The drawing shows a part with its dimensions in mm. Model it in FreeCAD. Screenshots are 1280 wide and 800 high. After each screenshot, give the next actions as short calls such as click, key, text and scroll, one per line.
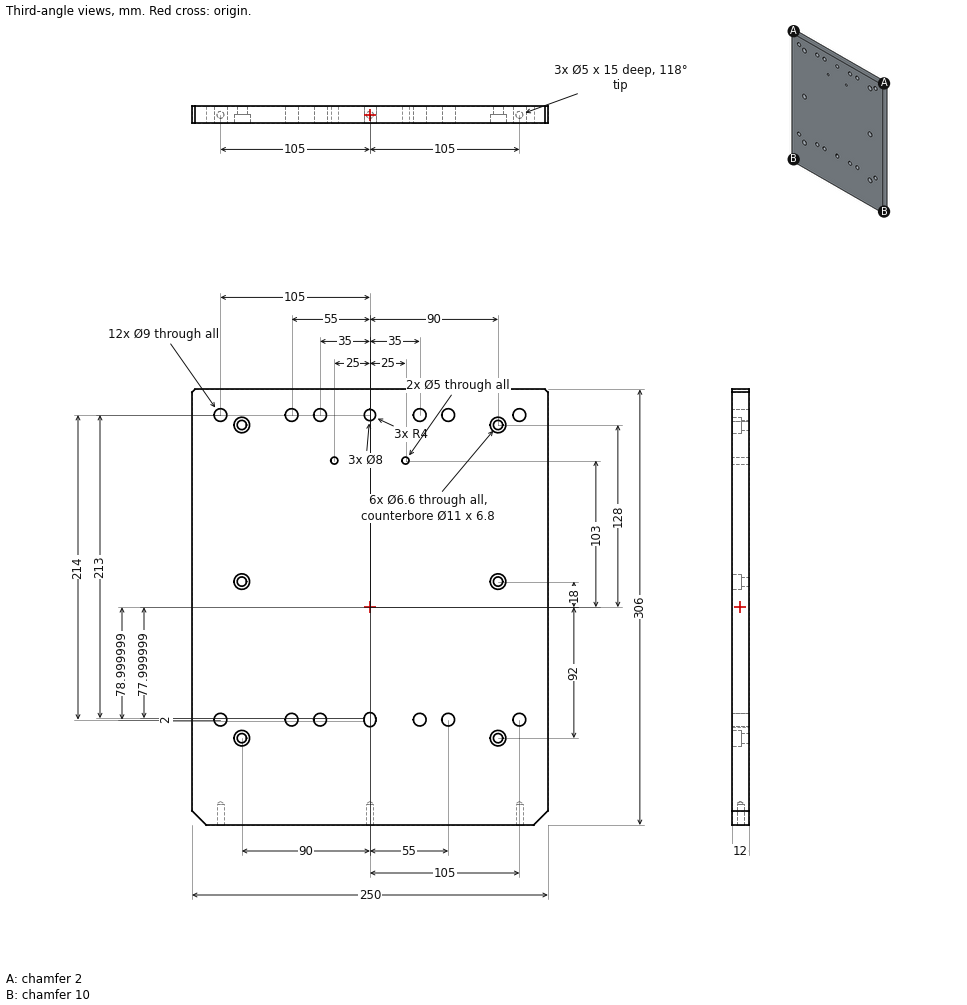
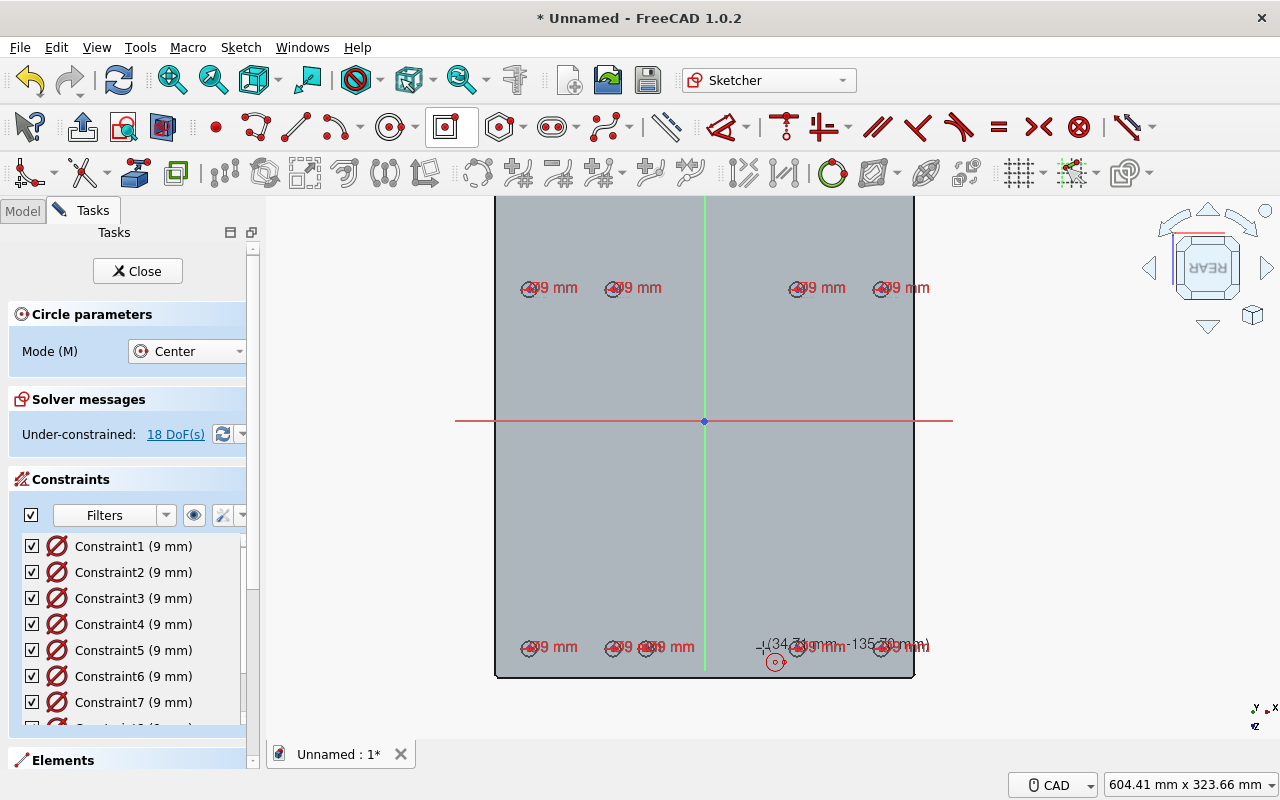
click(763, 648)
move(769, 642)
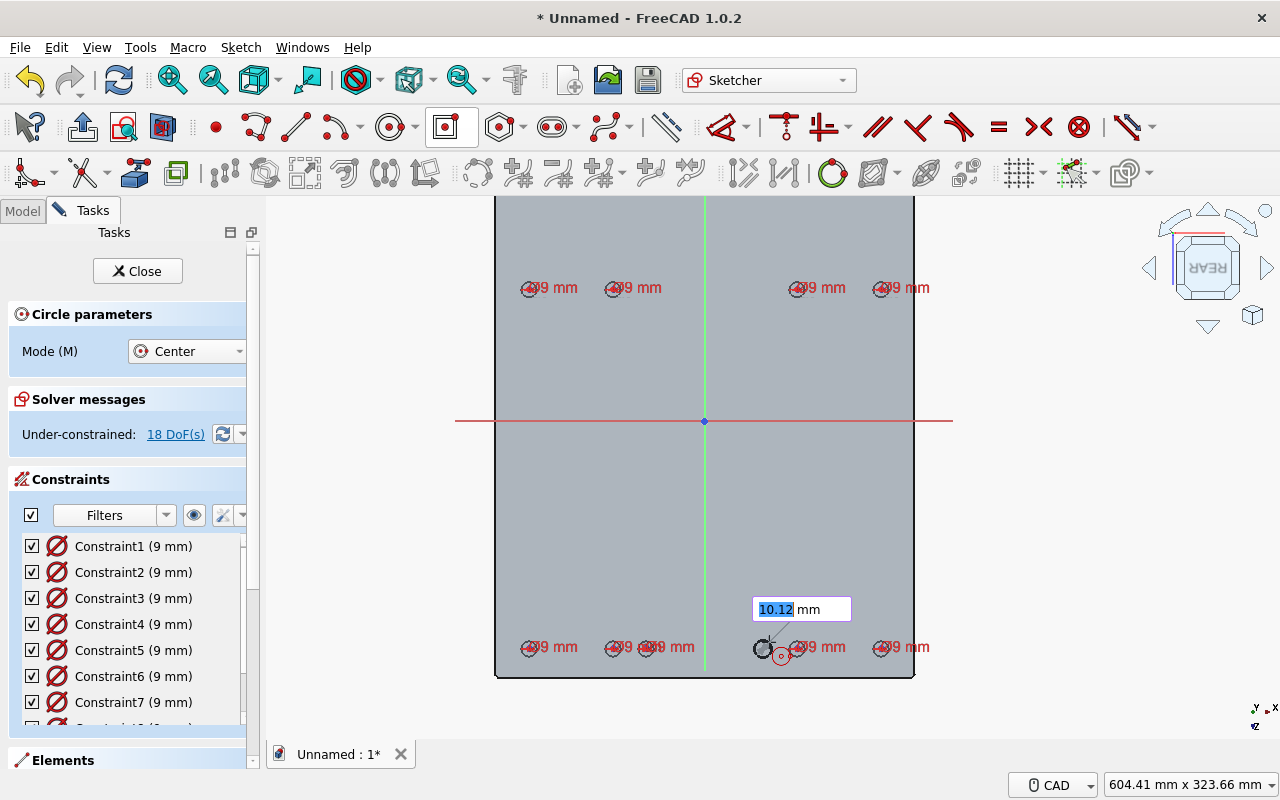
text(9)
key(Return)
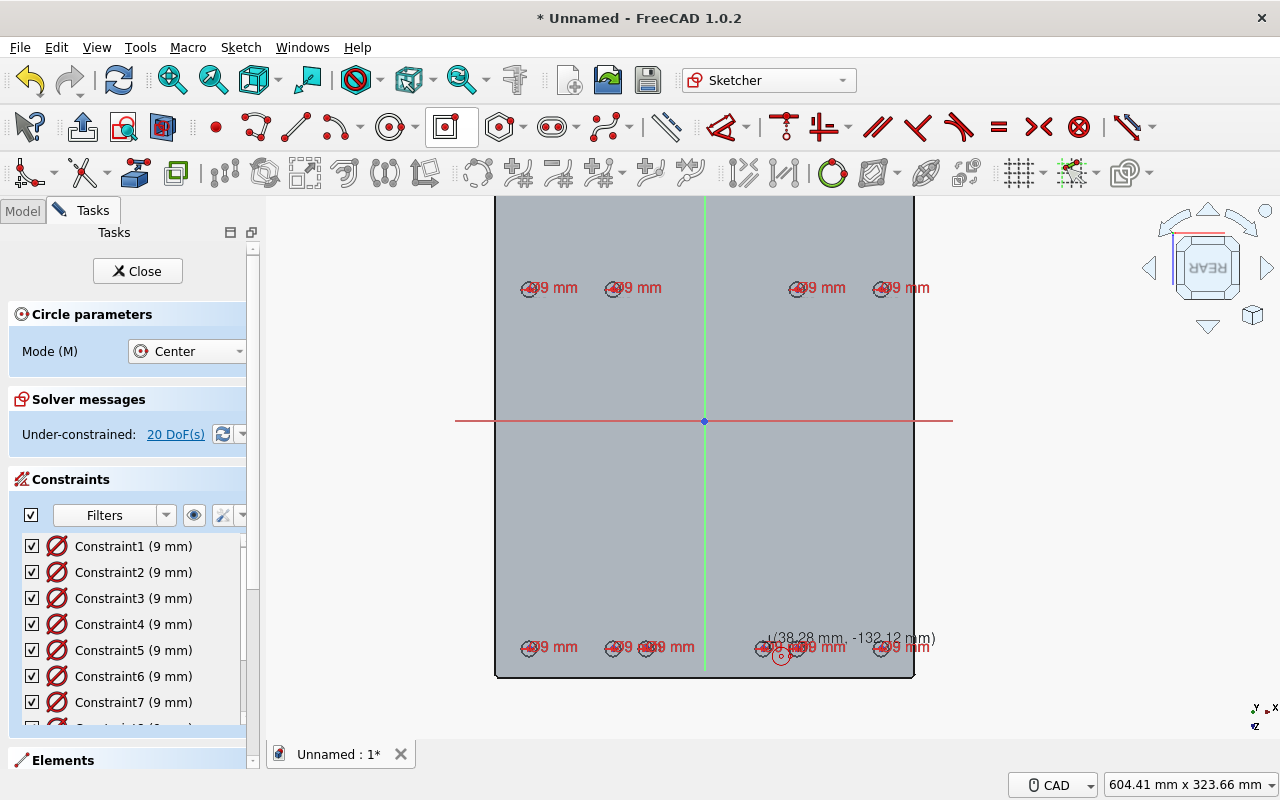
scroll(646, 289, up, 6)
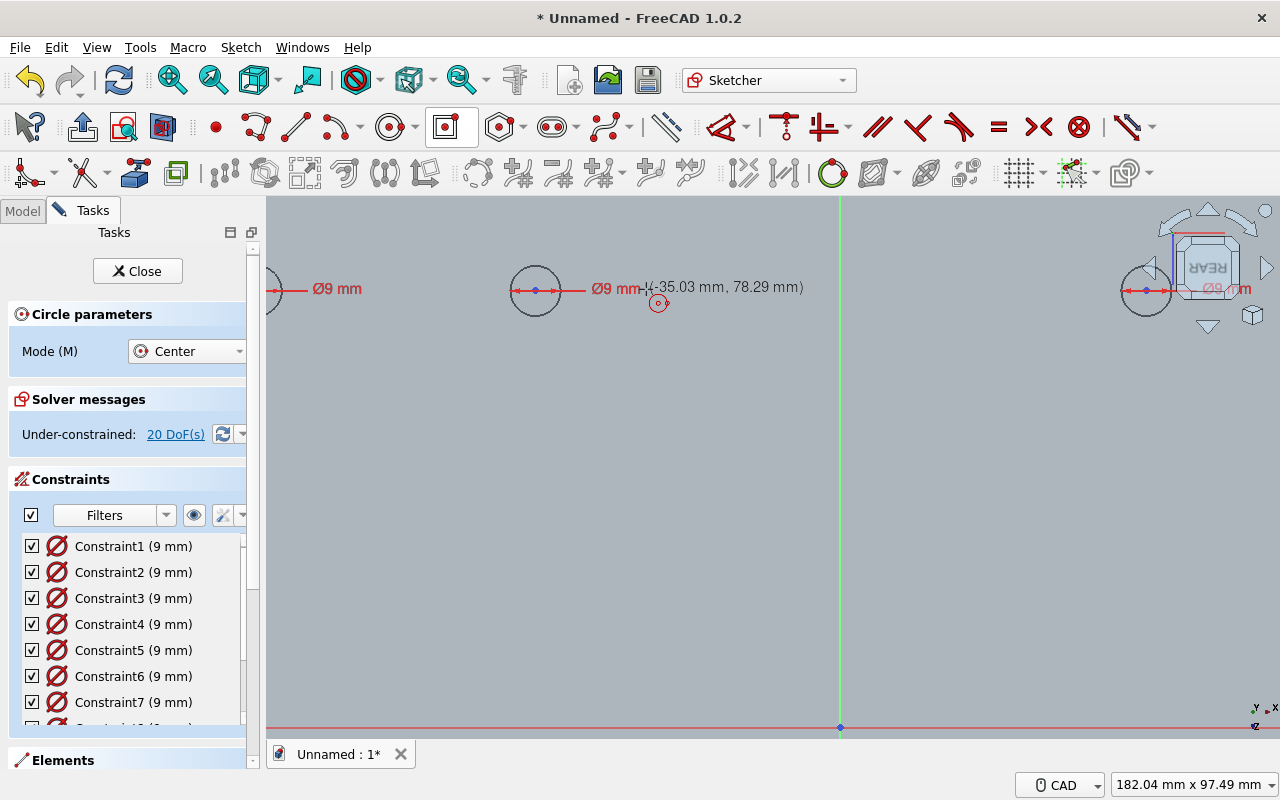
scroll(646, 288, down, 6)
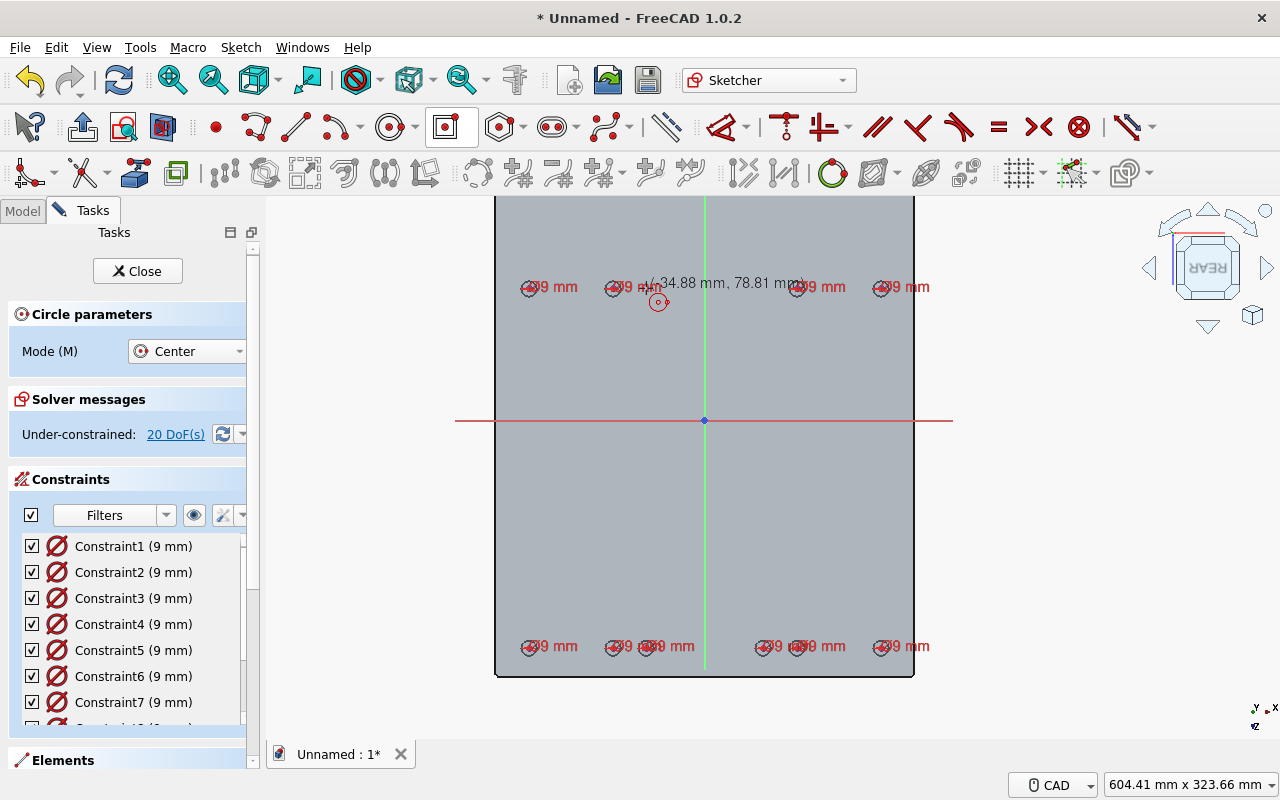
click(646, 288)
move(651, 283)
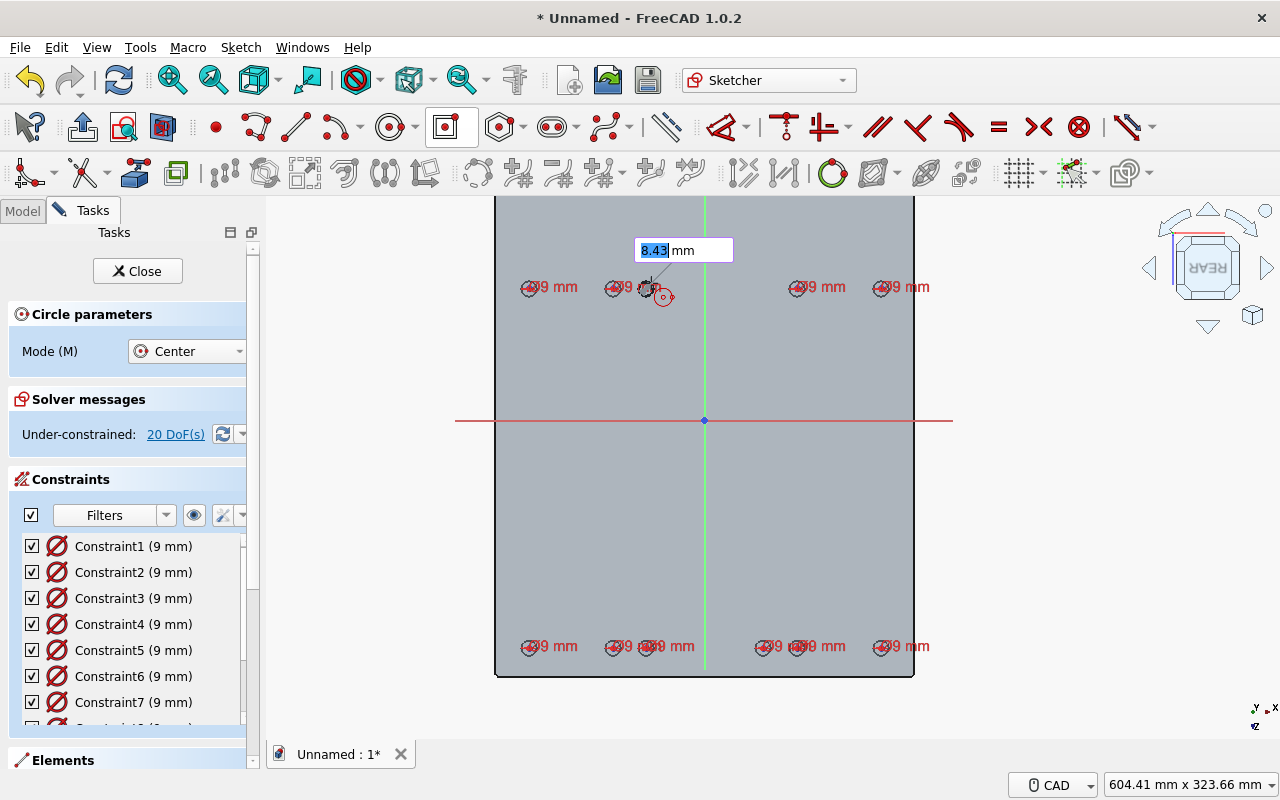
text(9)
key(Return)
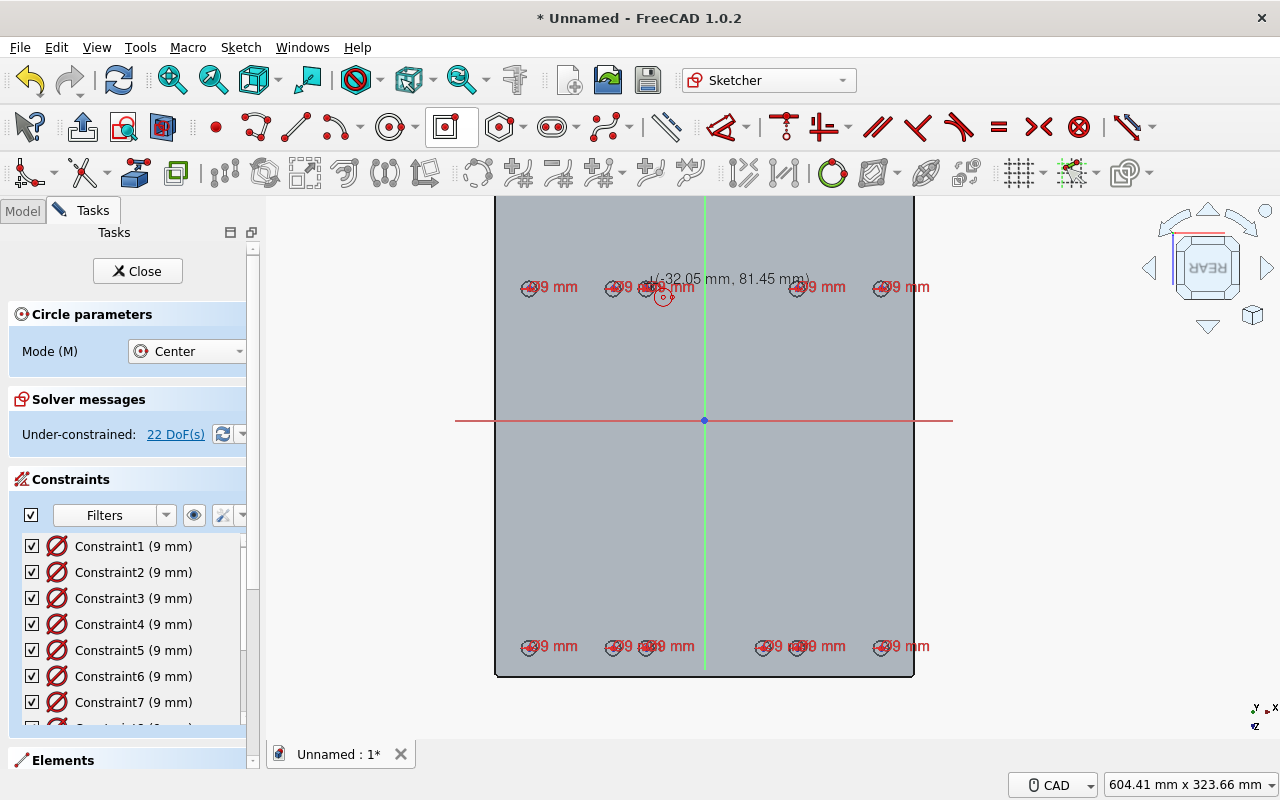
scroll(763, 288, up, 6)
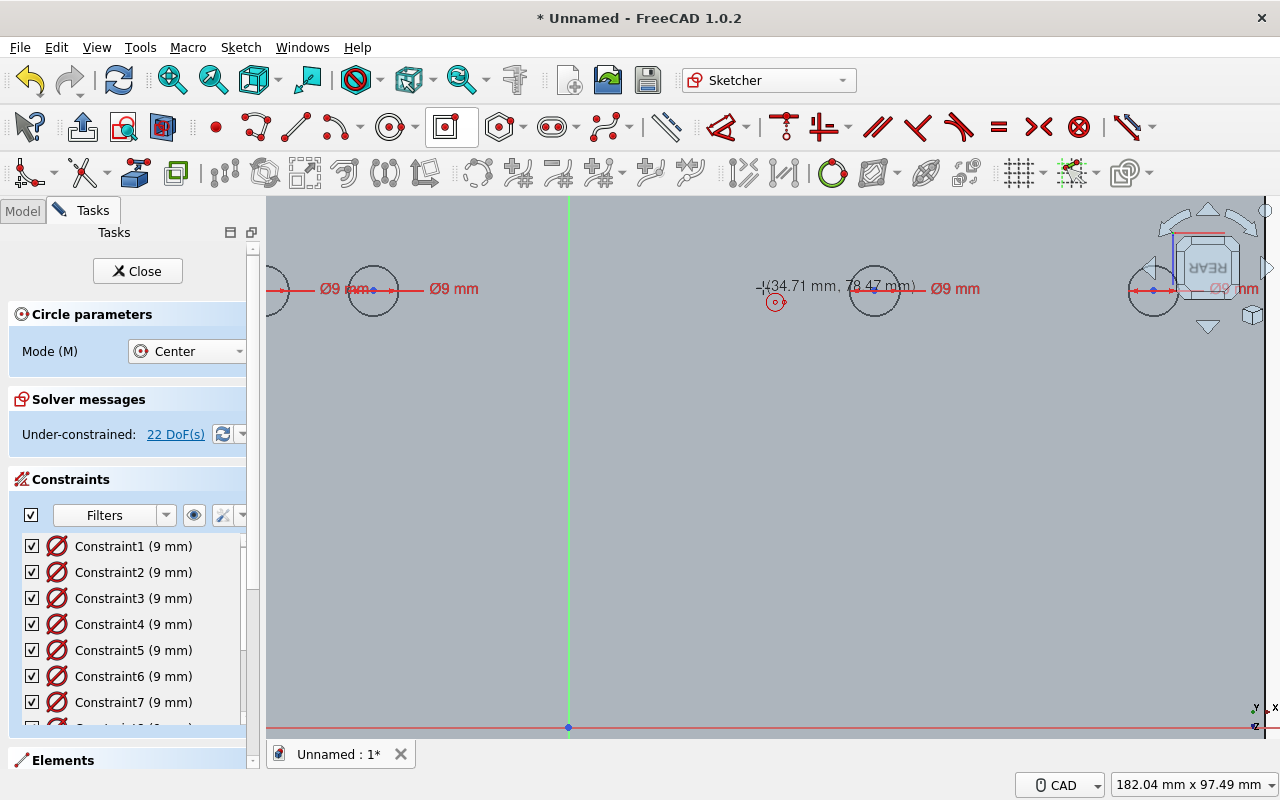
scroll(763, 288, down, 6)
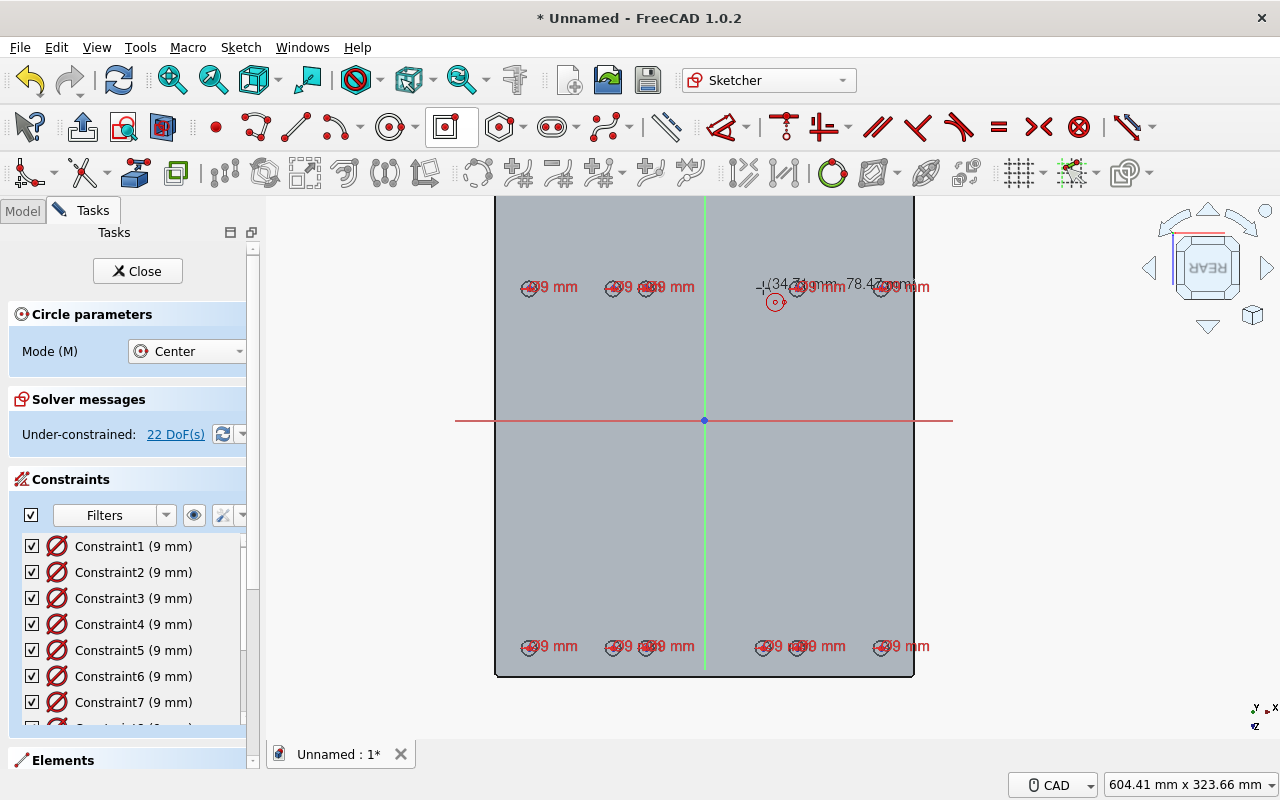
click(763, 288)
move(769, 283)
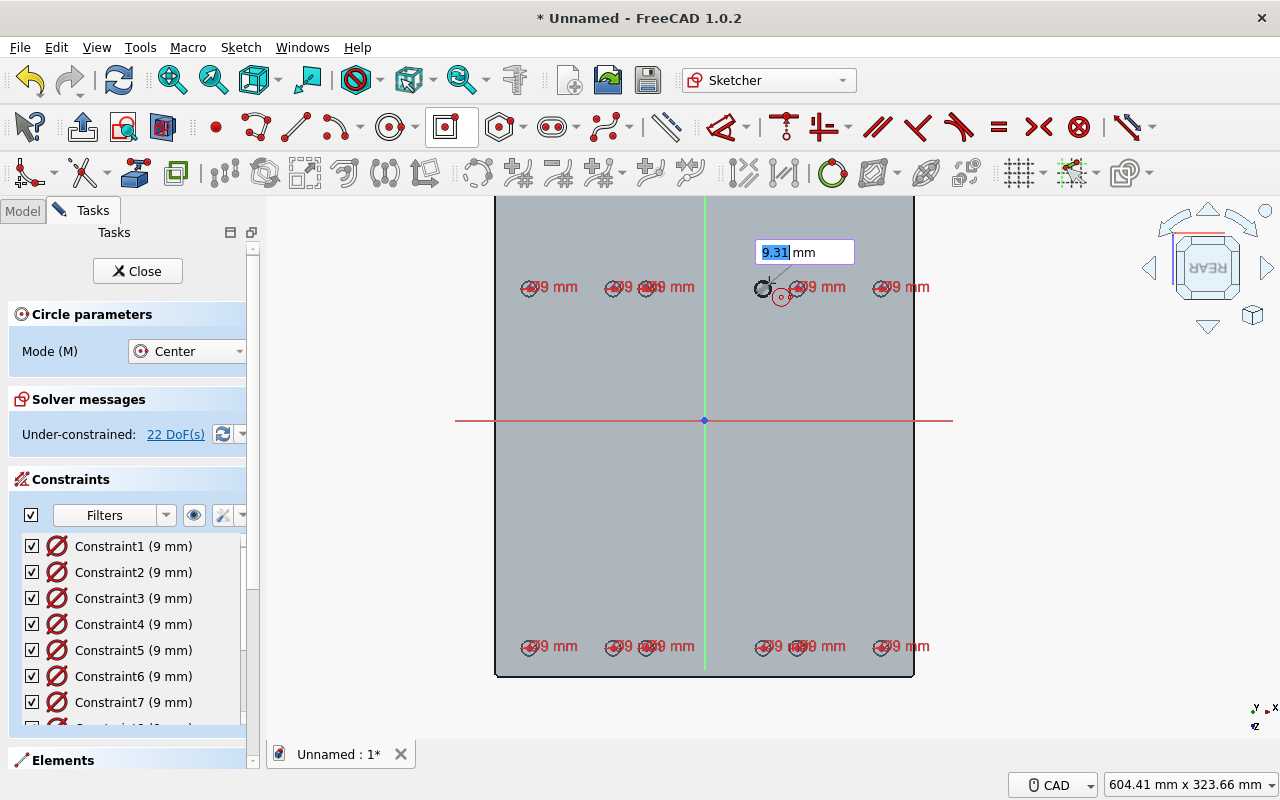
text(9)
key(Return)
key(Escape)